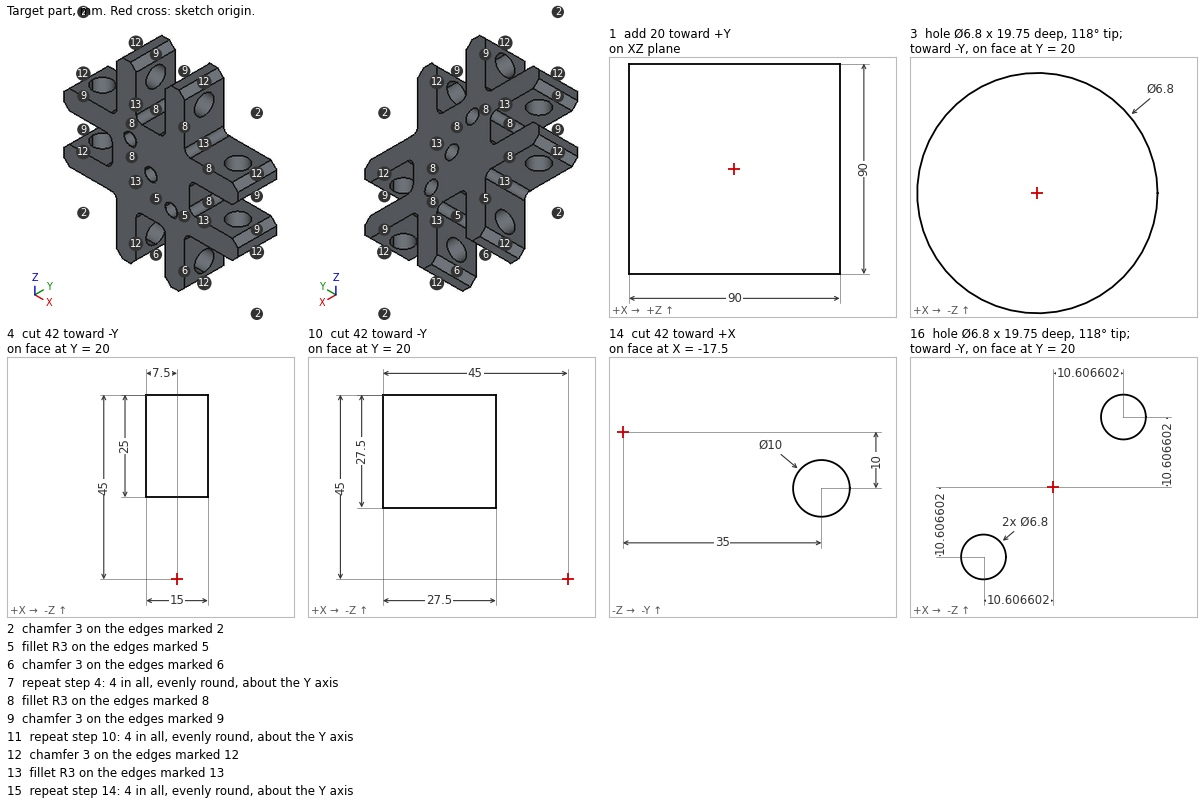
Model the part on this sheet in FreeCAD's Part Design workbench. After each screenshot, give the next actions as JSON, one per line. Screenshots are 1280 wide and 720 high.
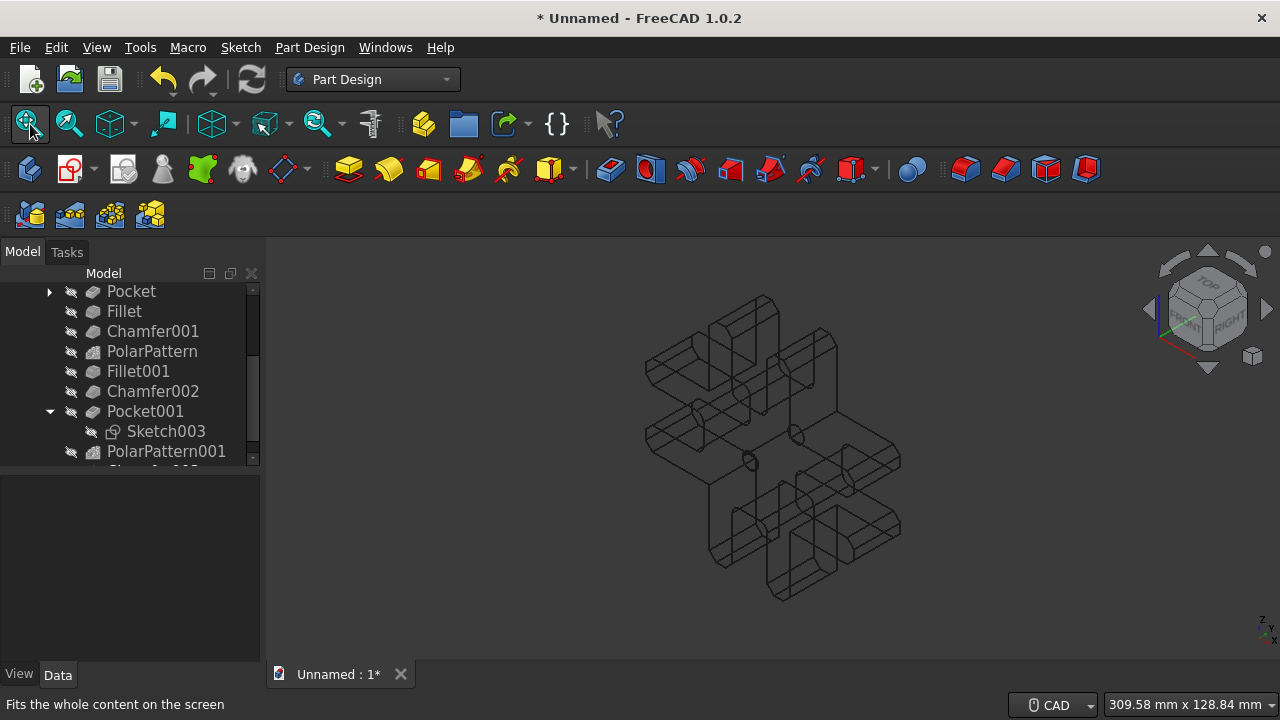
{"action": "left_click", "coordinate": [732, 470]}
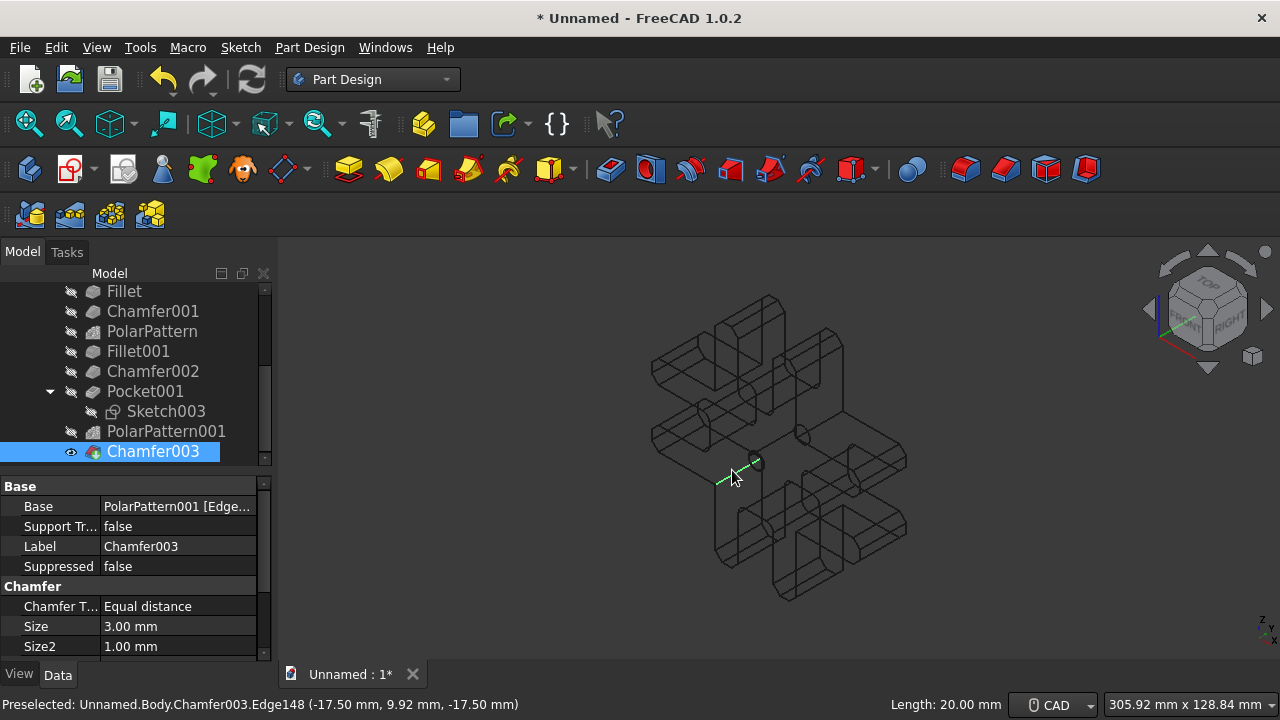
{"action": "left_click", "coordinate": [748, 371], "text": "ctrl"}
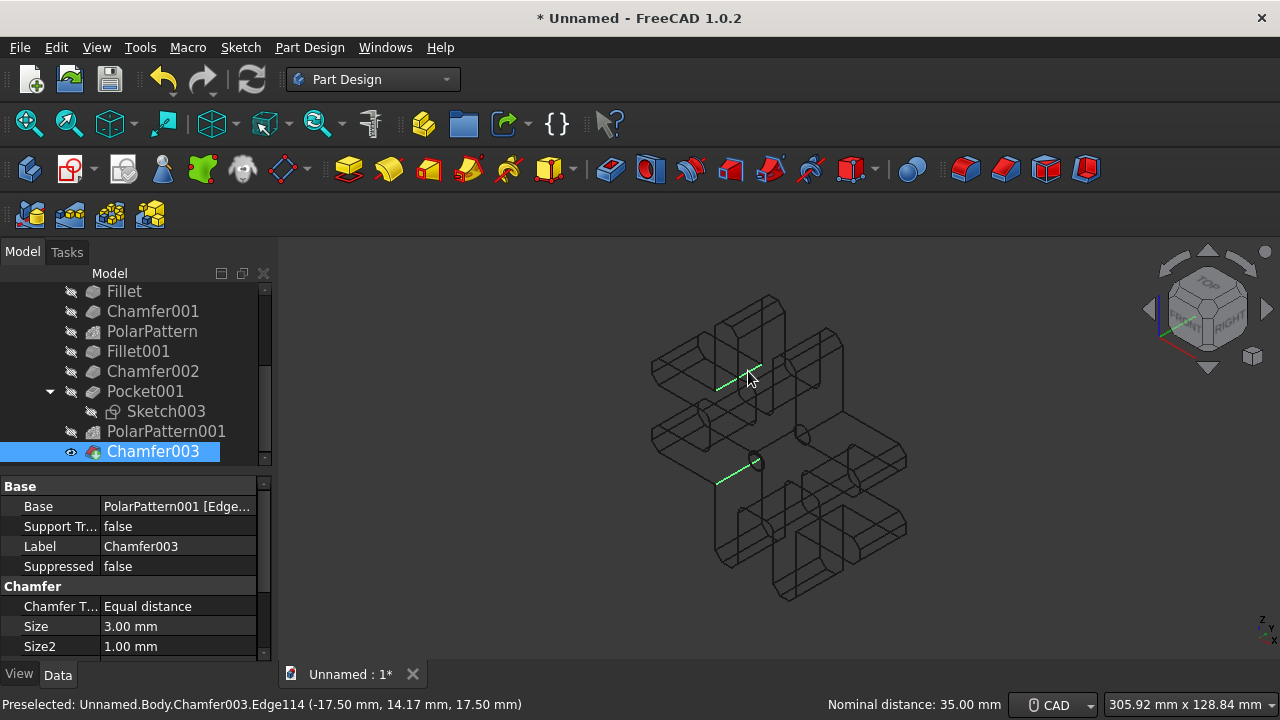
{"action": "left_click", "coordinate": [820, 424], "text": "ctrl"}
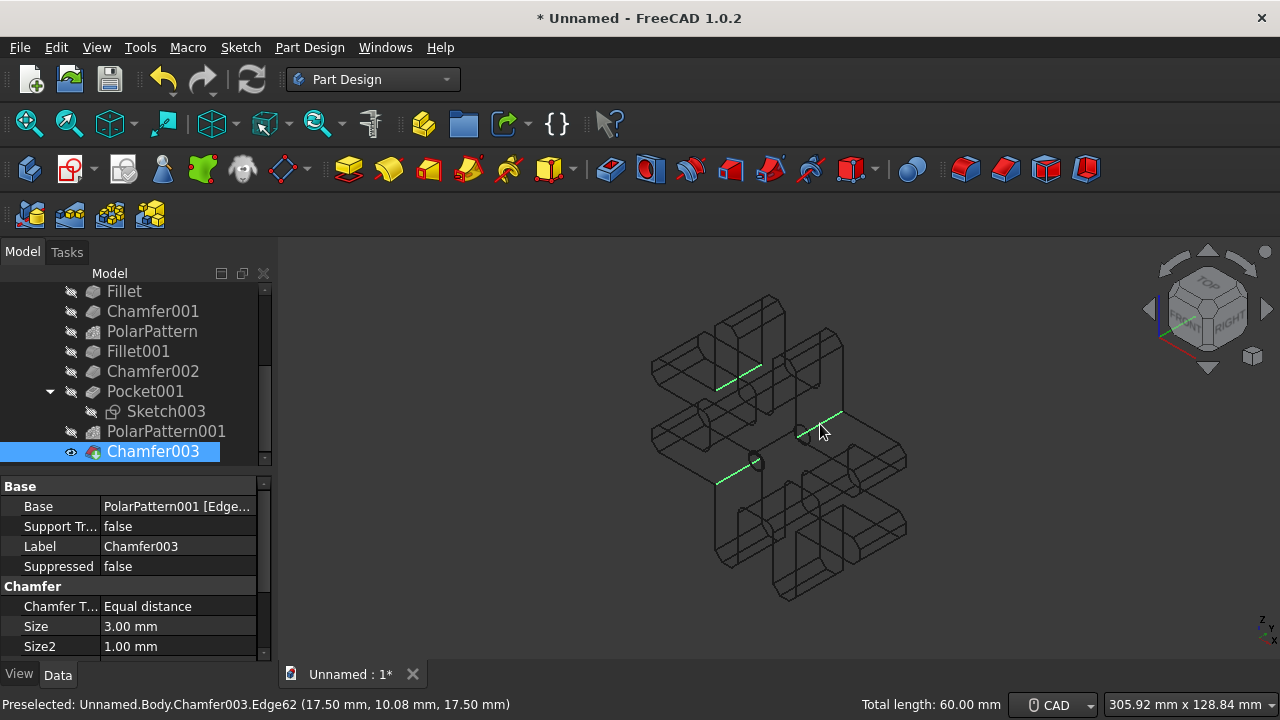
{"action": "left_click", "coordinate": [829, 512], "text": "ctrl"}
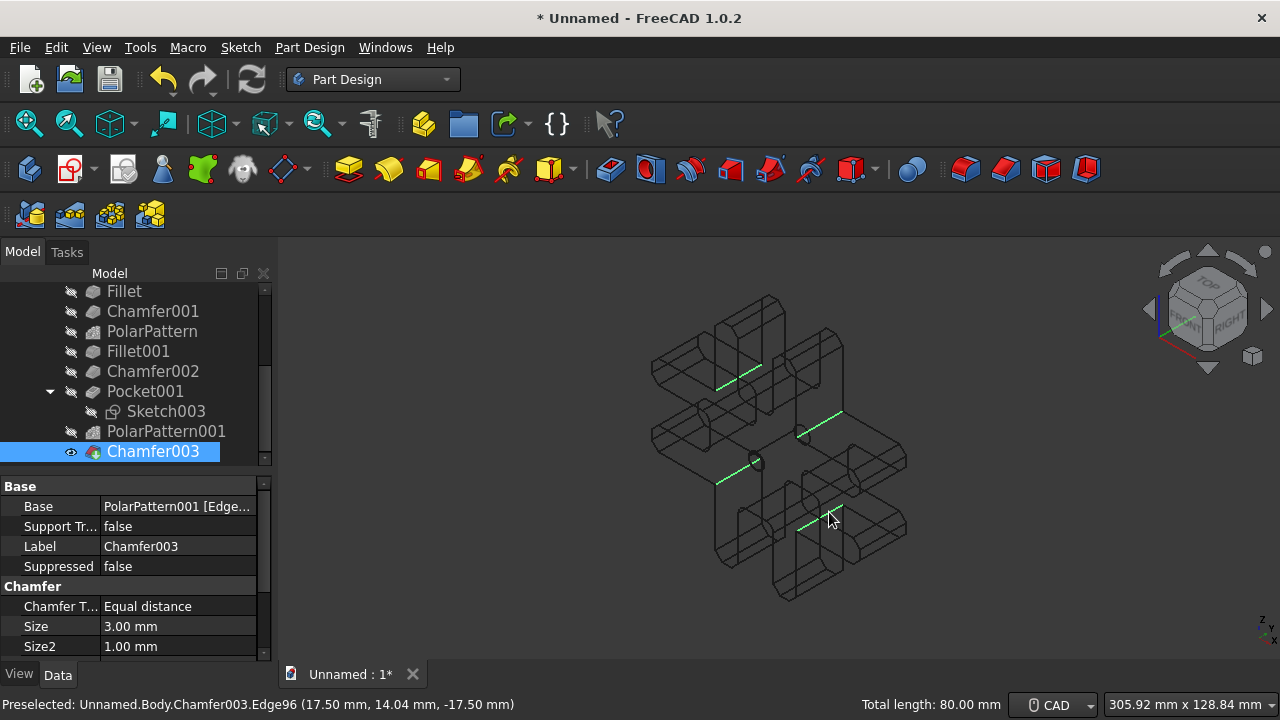
{"action": "key", "text": "v 1"}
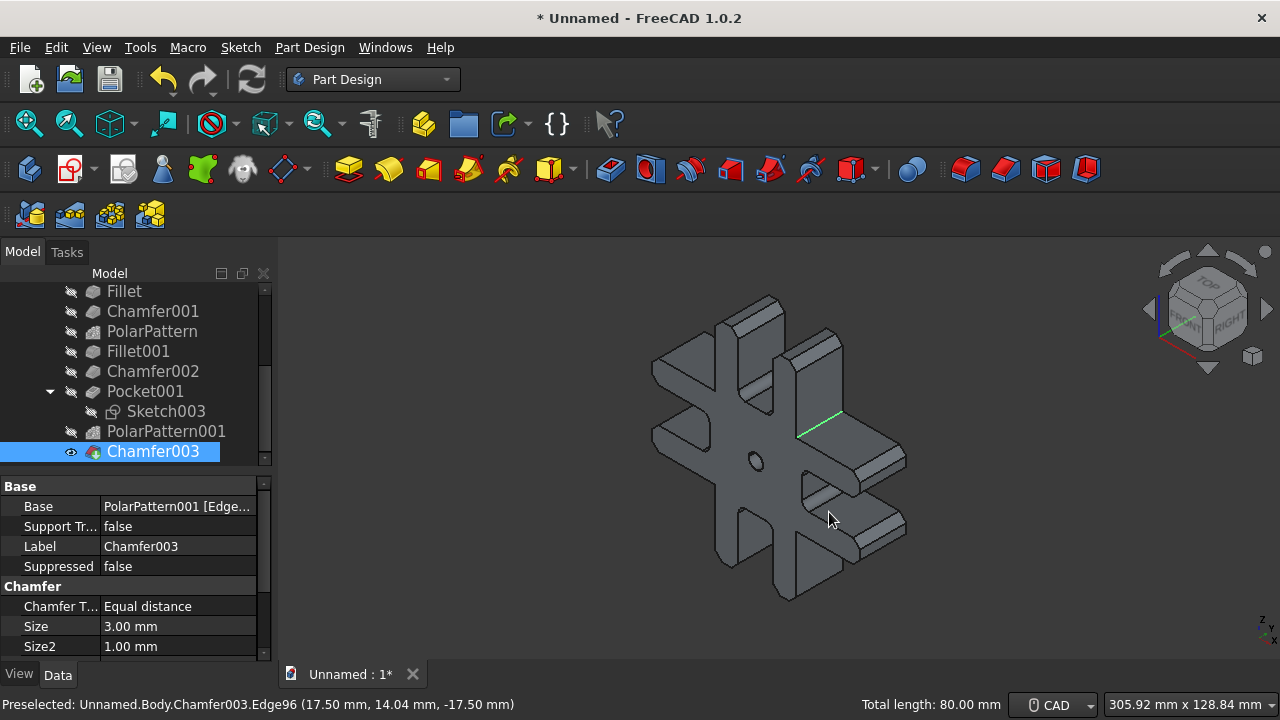
{"action": "left_click", "coordinate": [966, 170]}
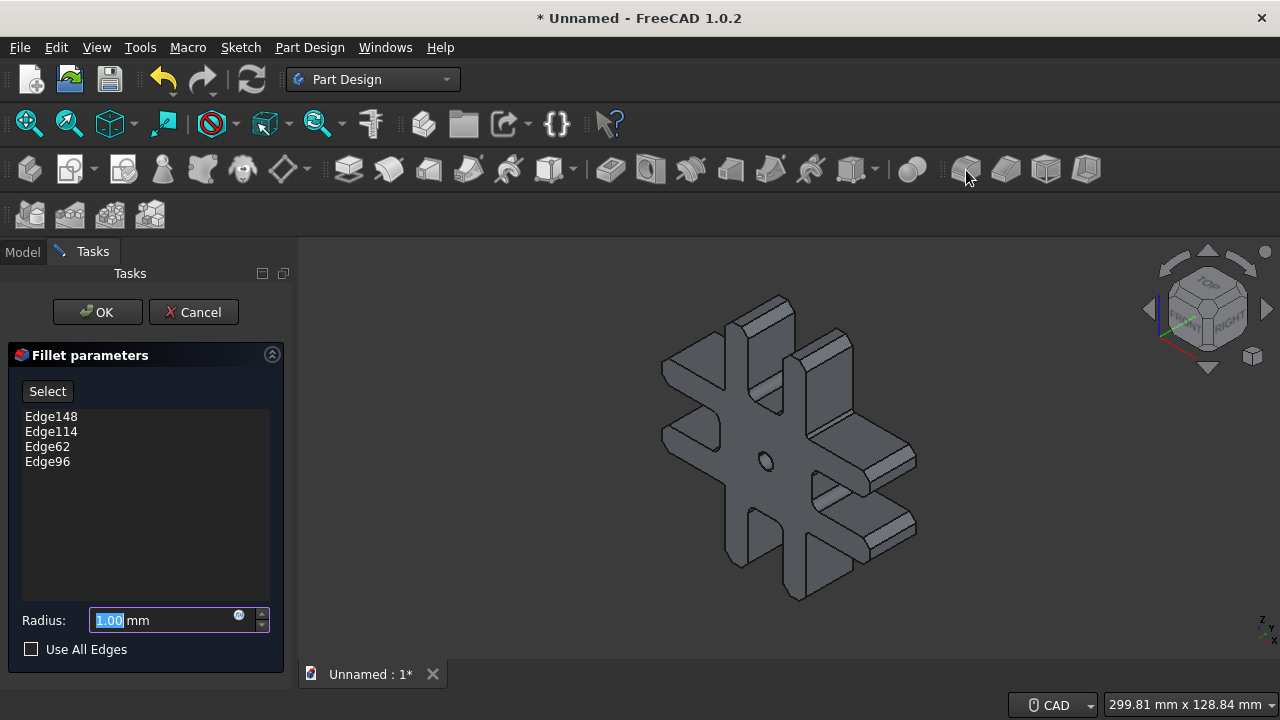
{"action": "type", "text": "3"}
{"action": "key", "text": "Tab"}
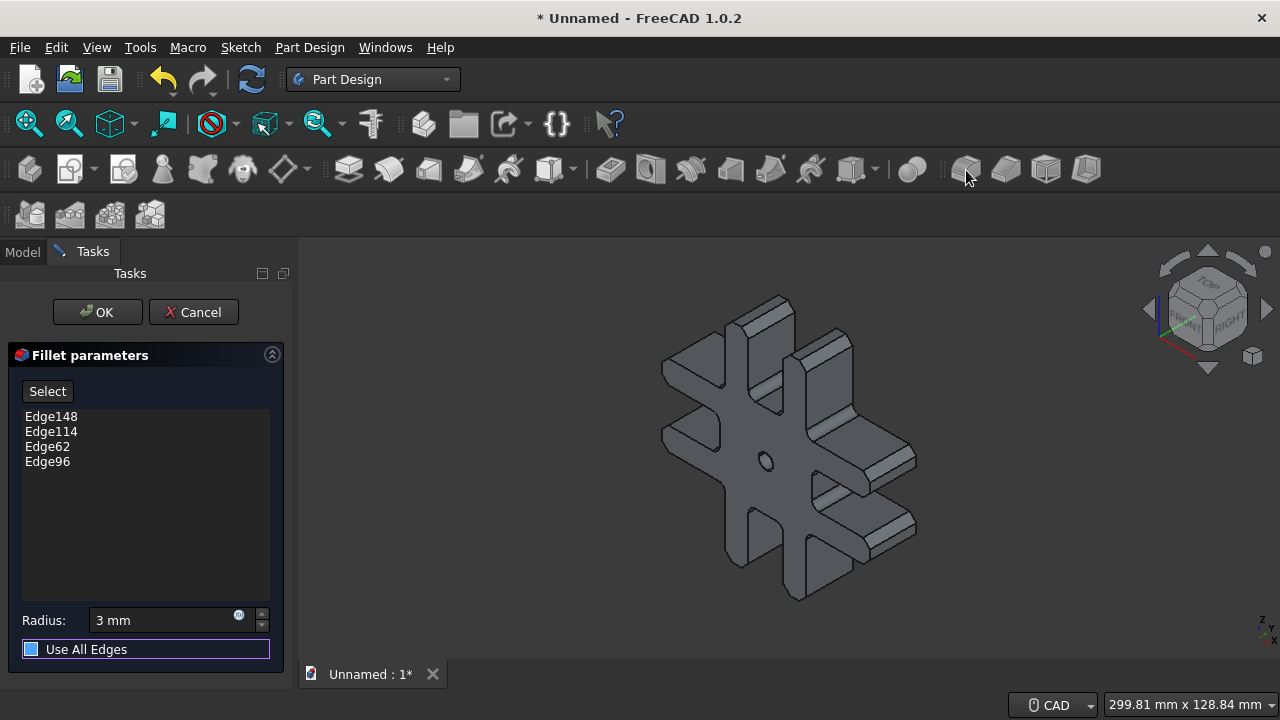
{"action": "left_click", "coordinate": [98, 312]}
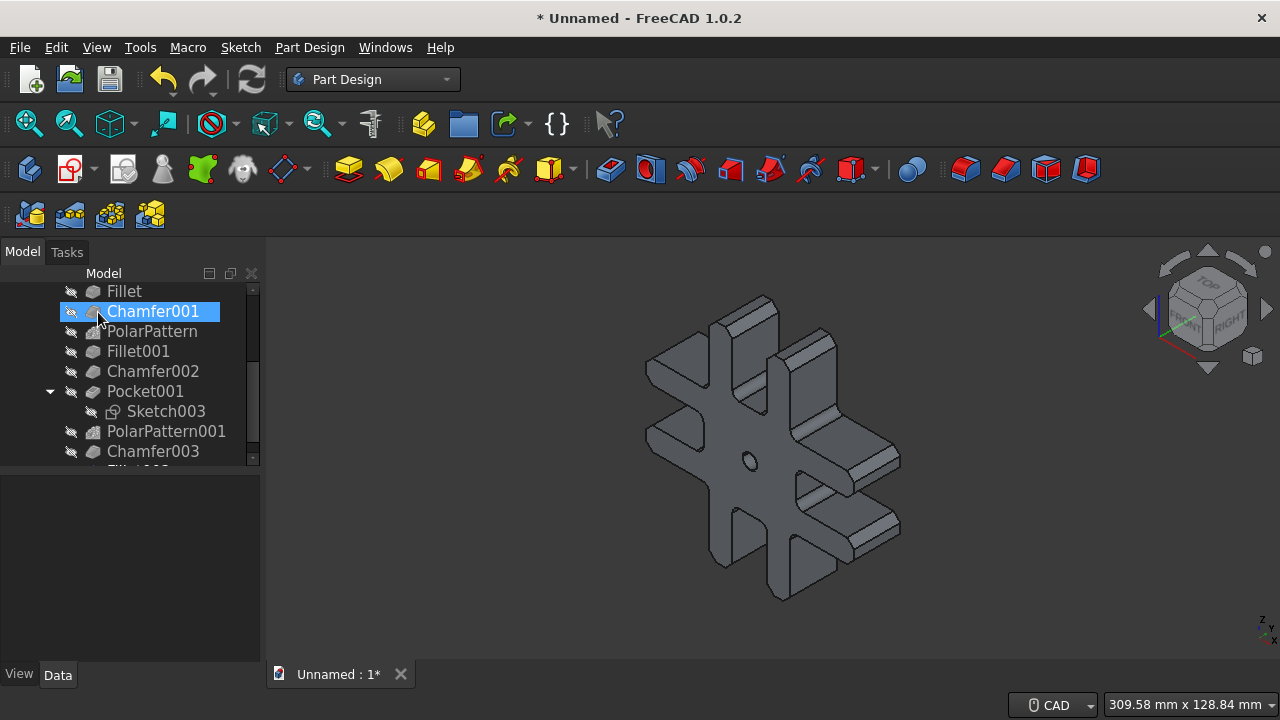
{"action": "key", "text": "6"}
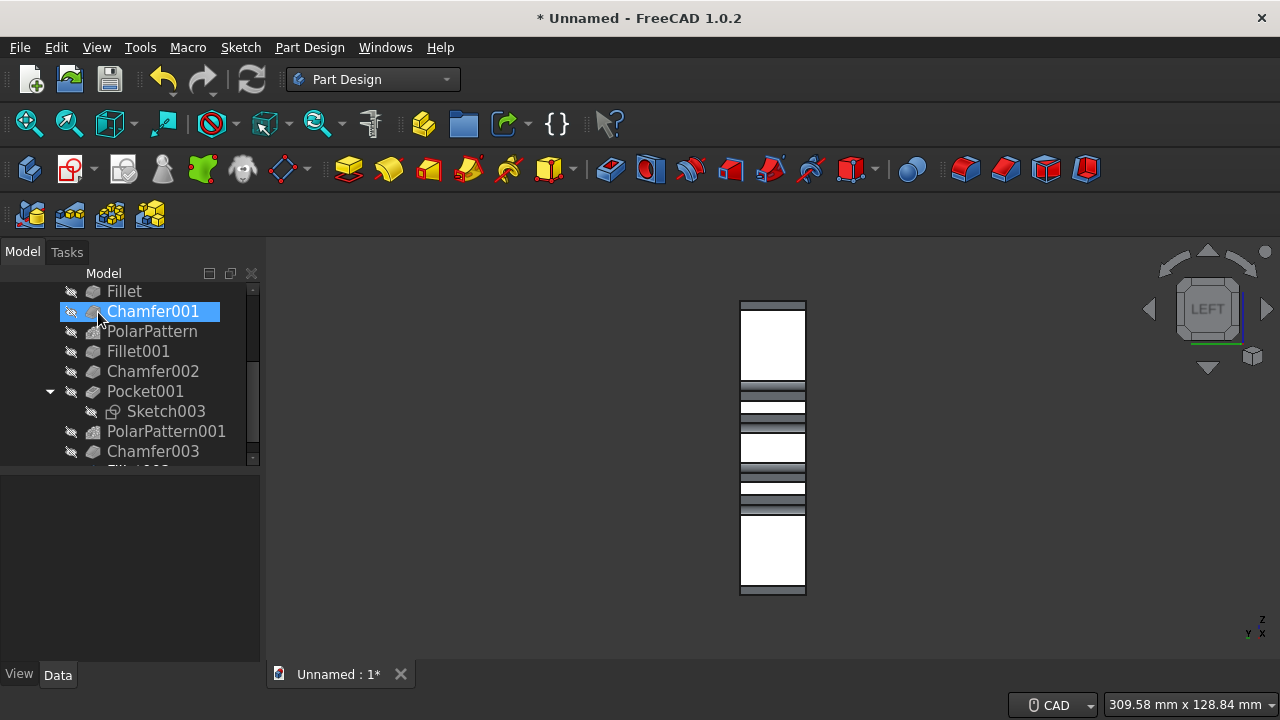
{"action": "left_click", "coordinate": [773, 549]}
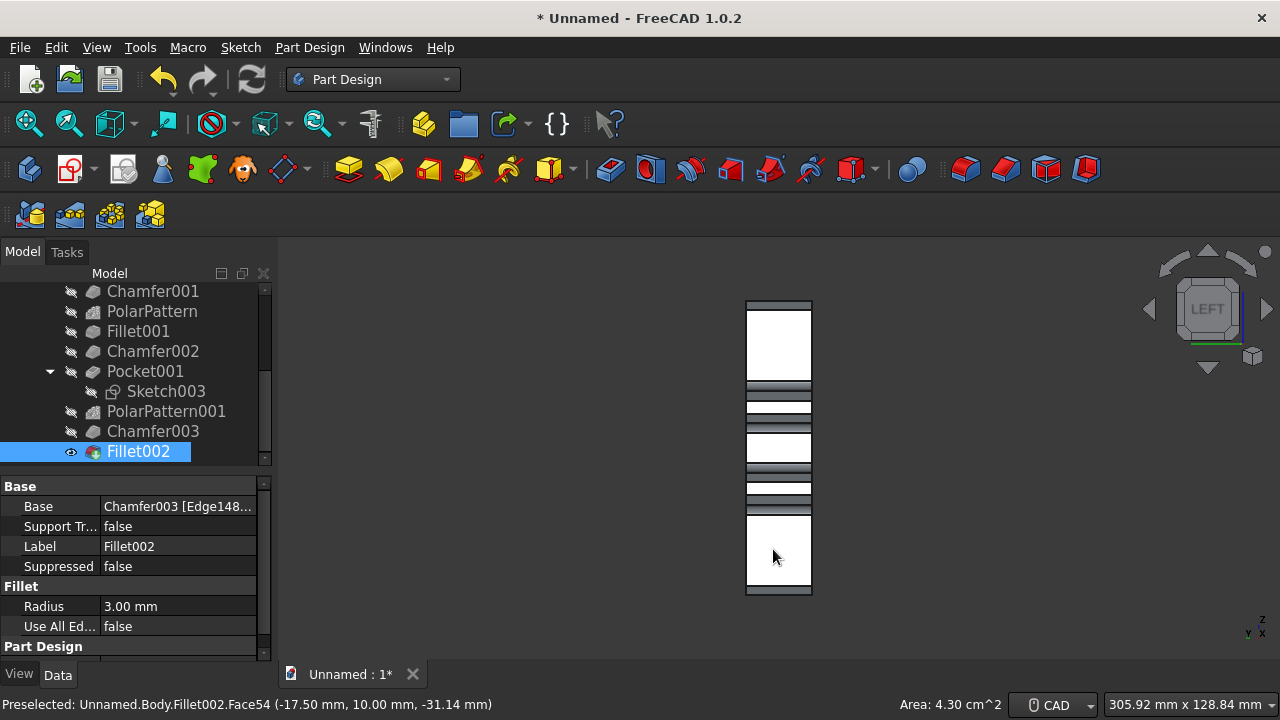
{"action": "left_click", "coordinate": [70, 170]}